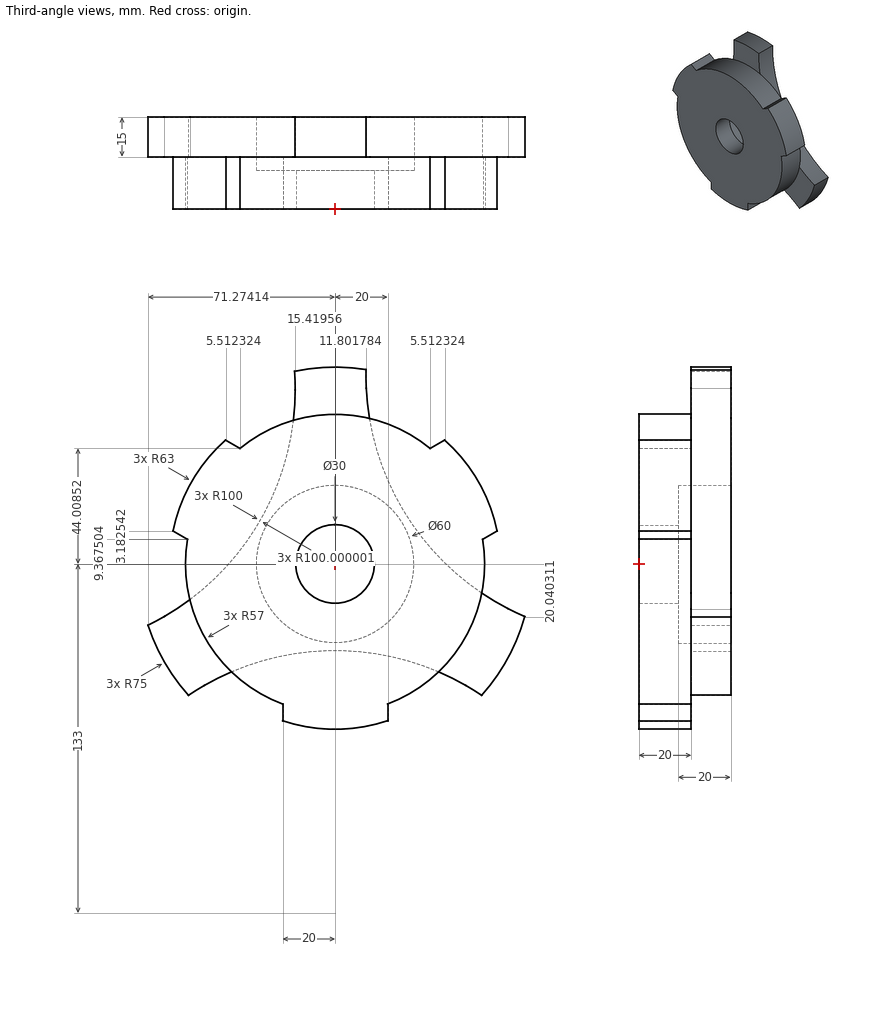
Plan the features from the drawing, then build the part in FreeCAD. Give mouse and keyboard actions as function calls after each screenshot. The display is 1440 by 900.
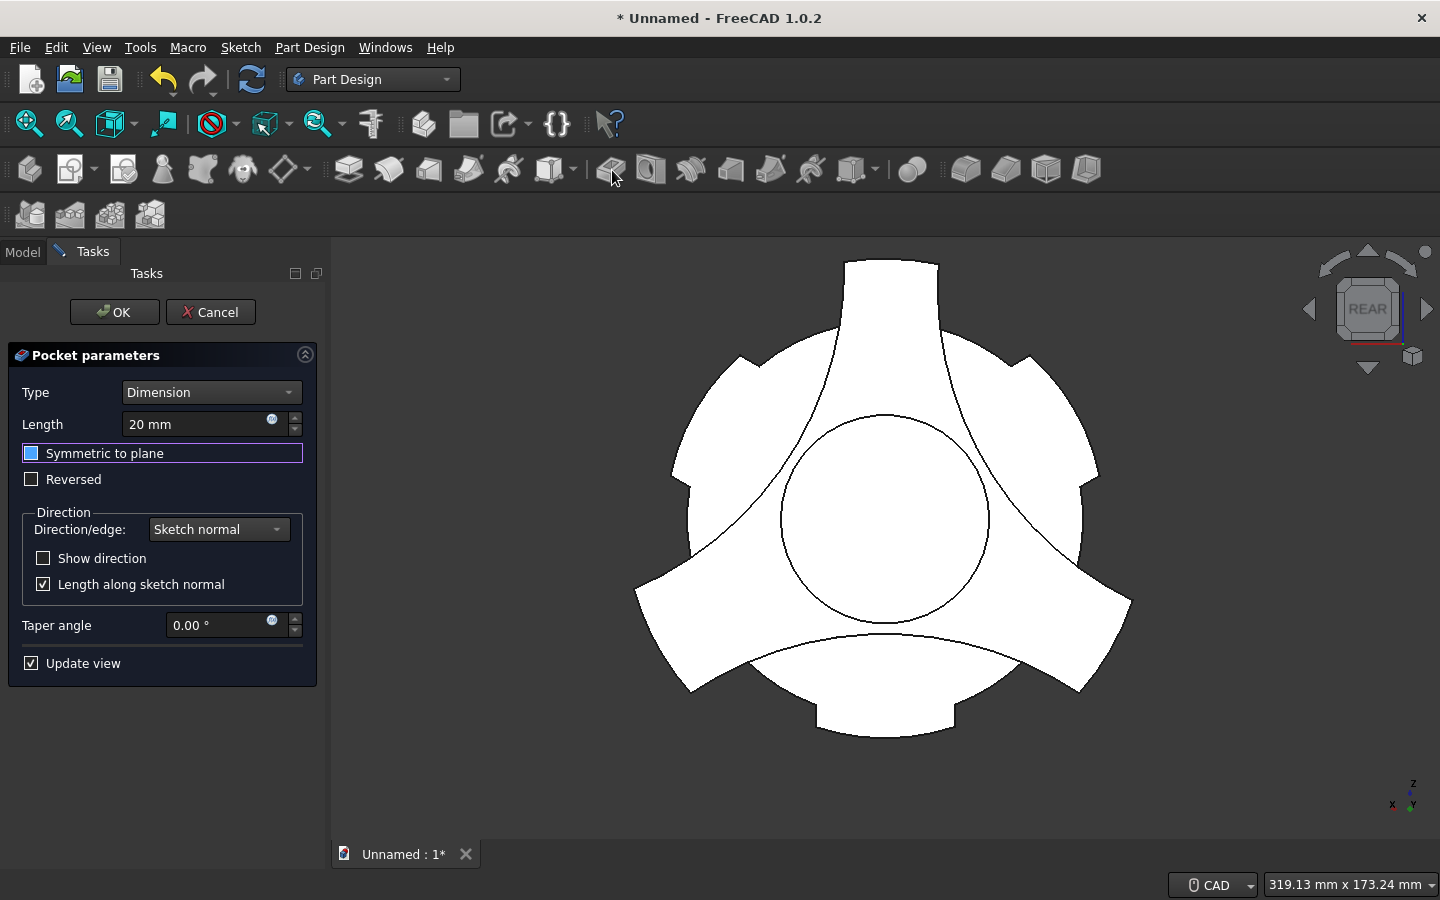
click(115, 312)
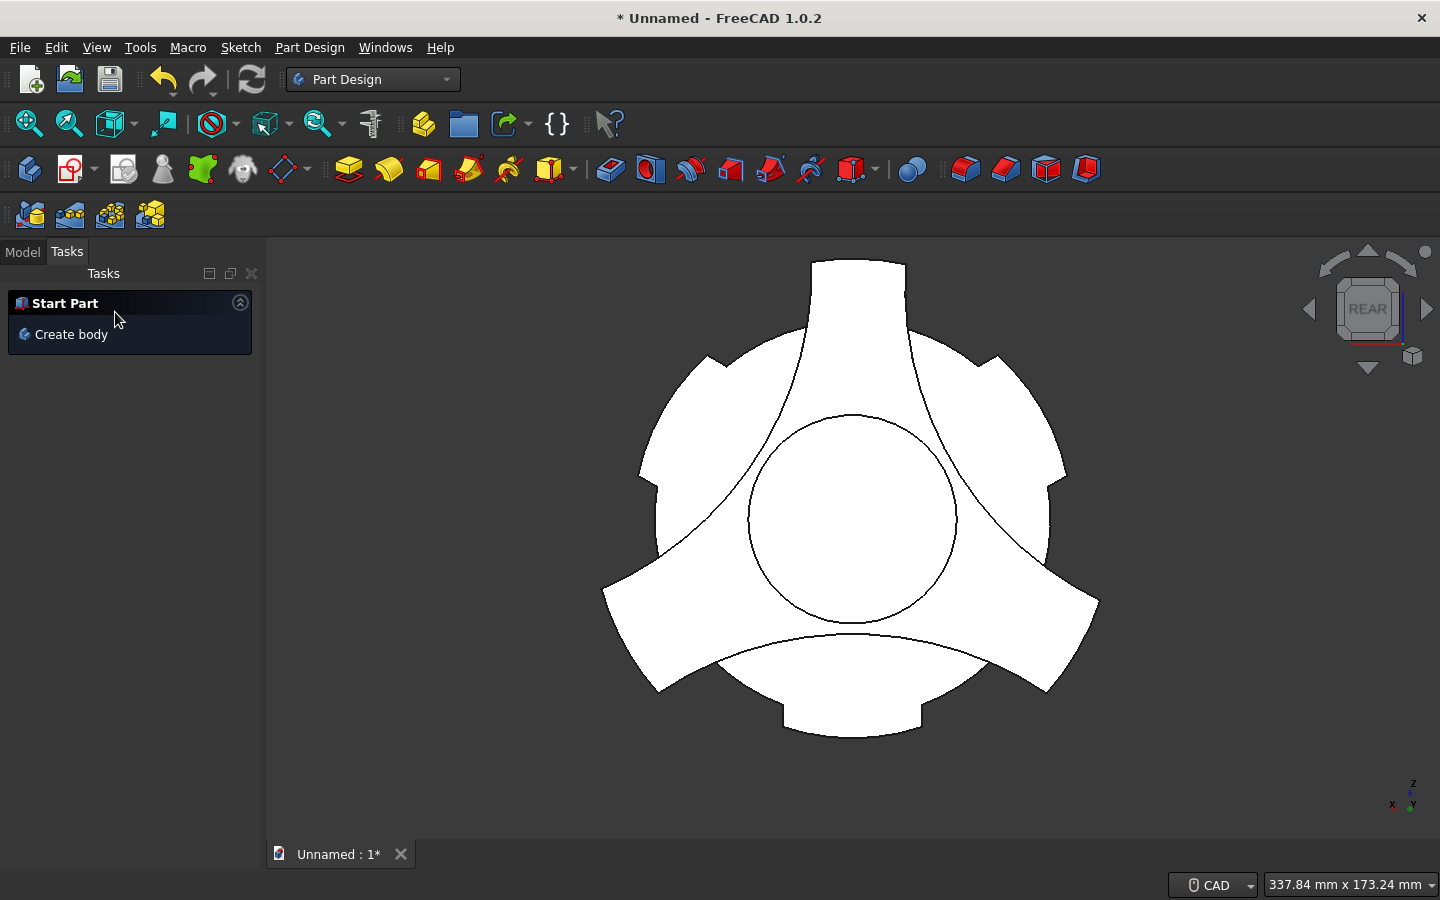
click(853, 518)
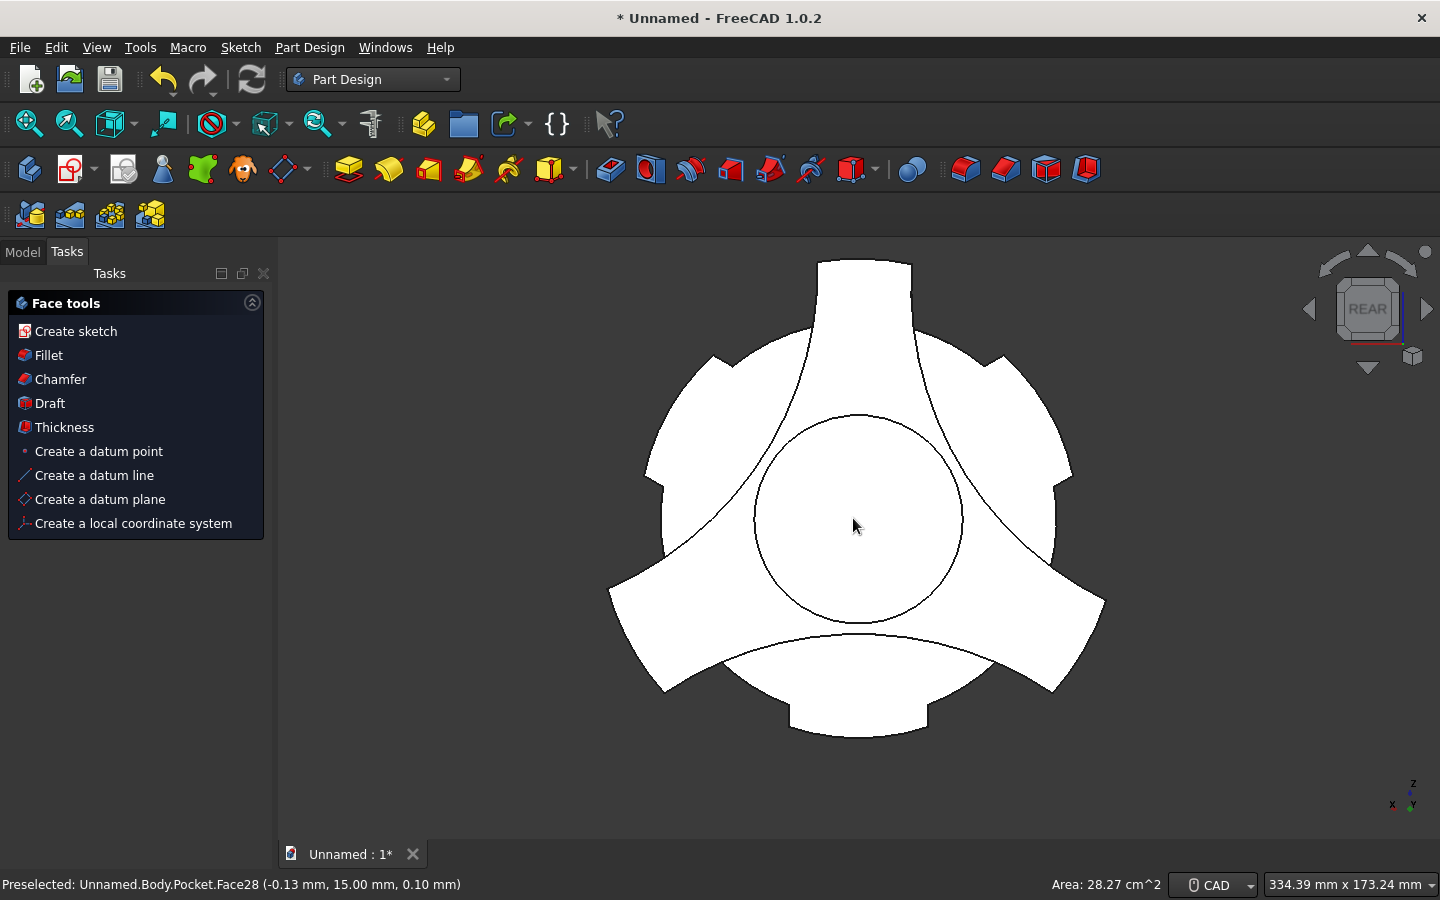
click(70, 170)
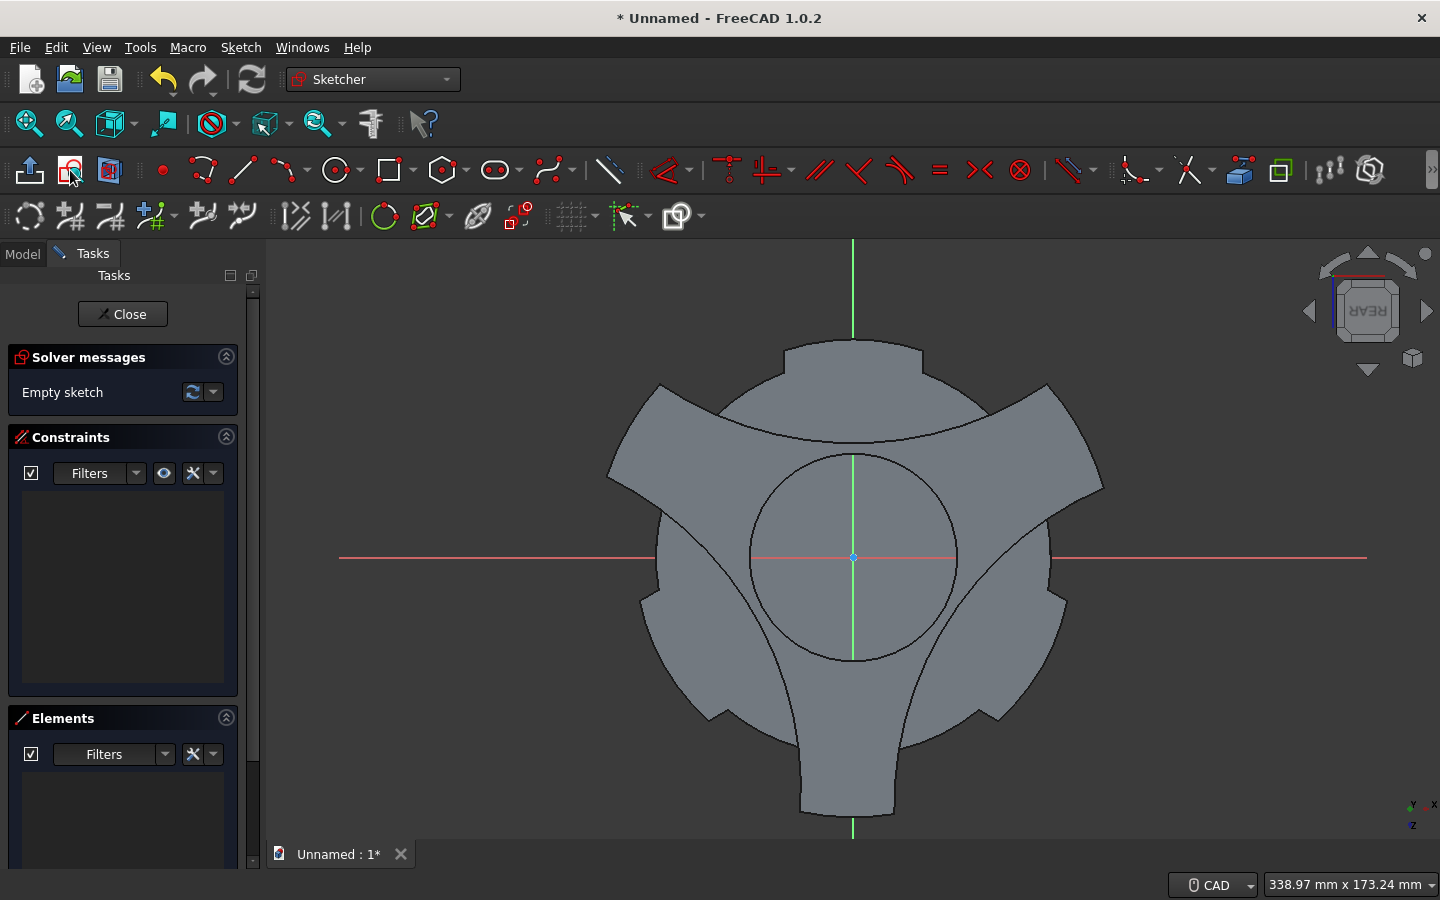
click(110, 170)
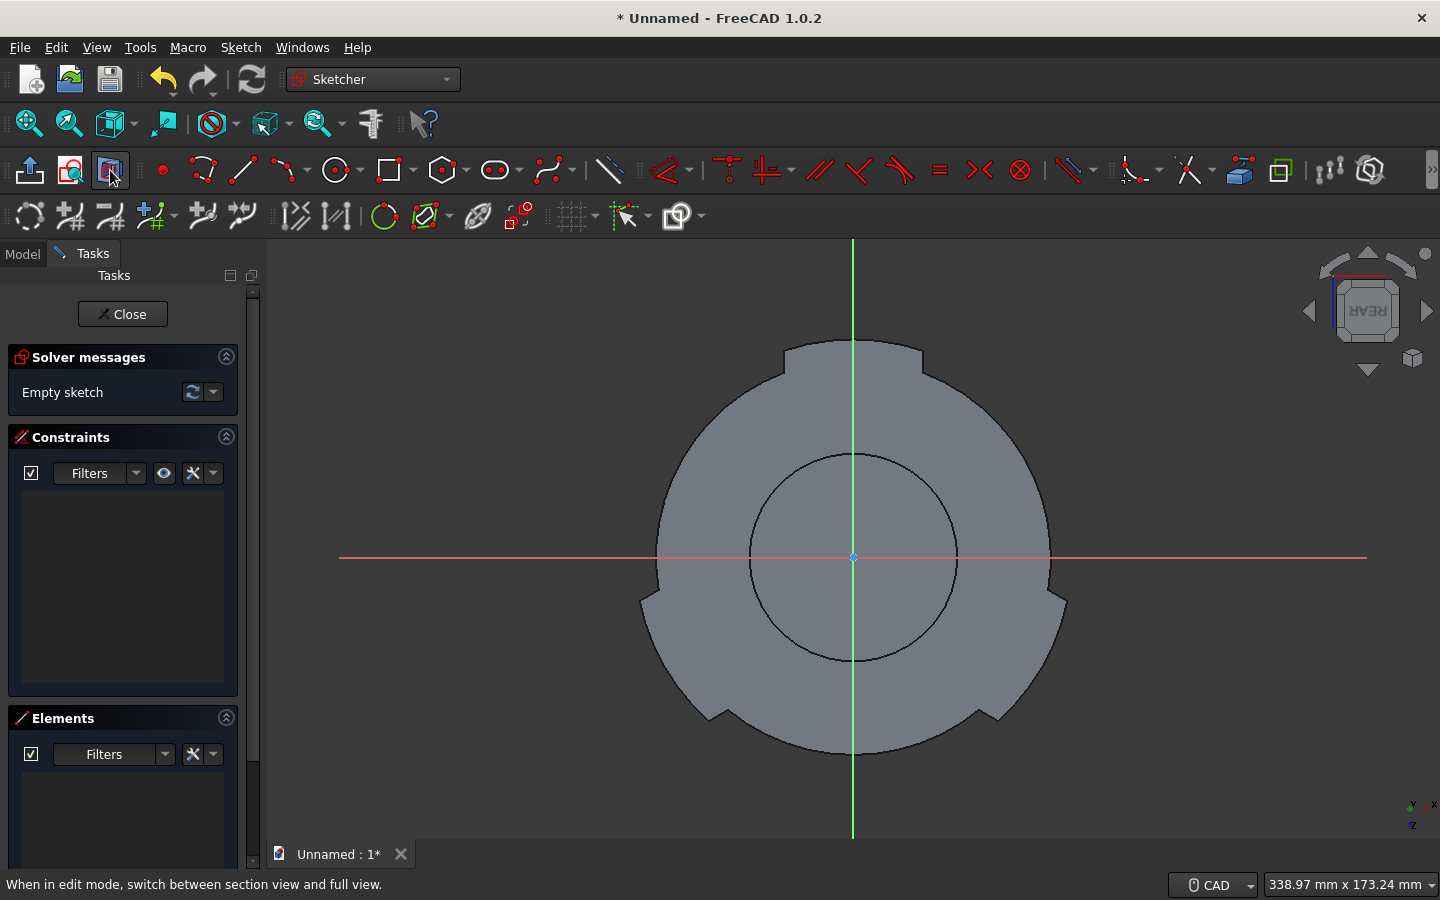
scroll(876, 564, up, 7)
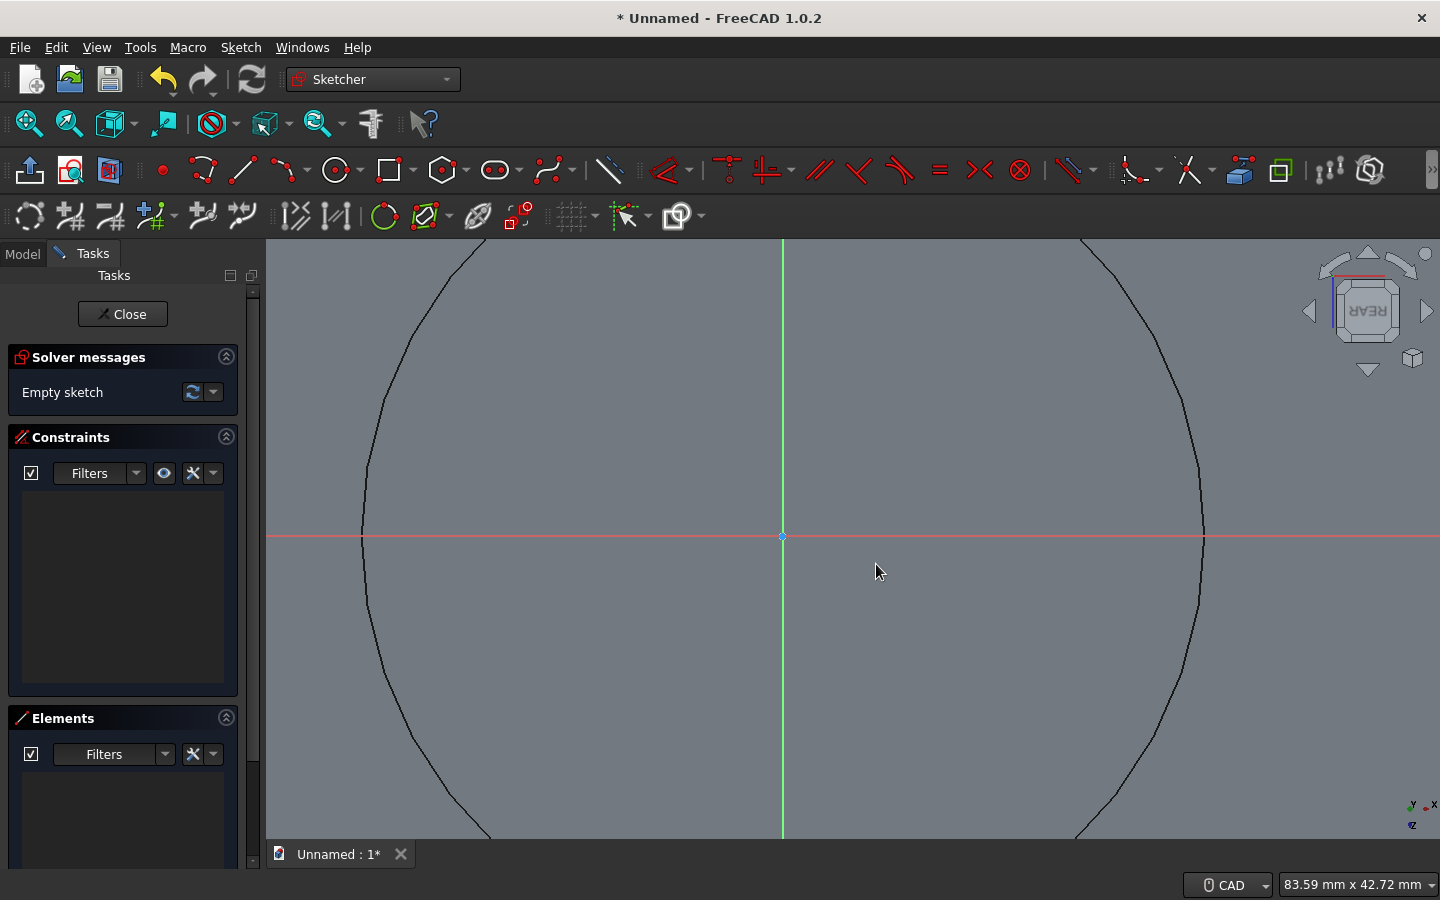
click(336, 170)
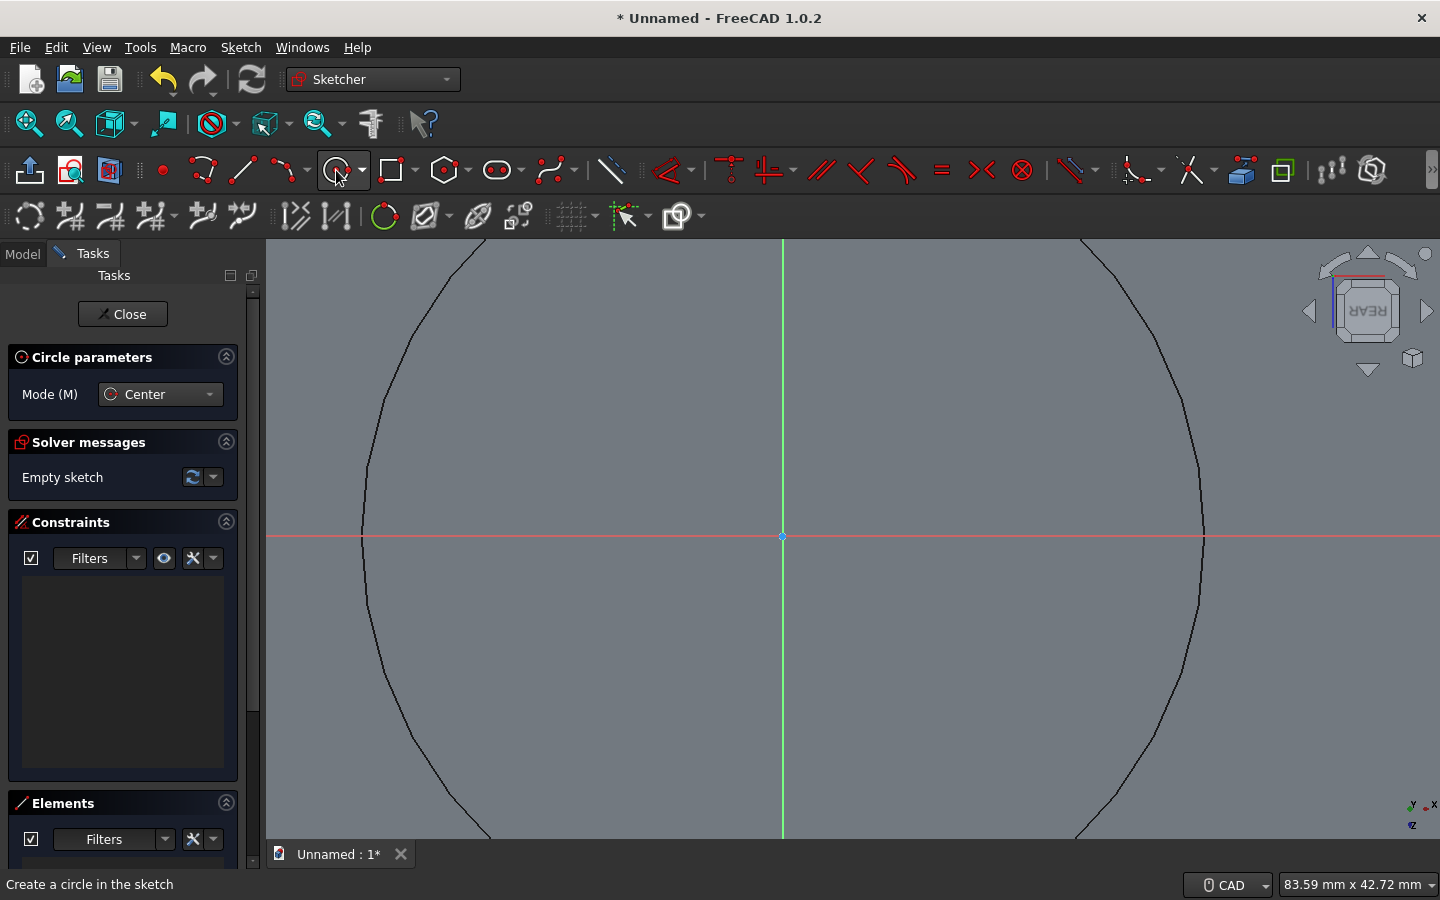
click(783, 536)
move(932, 387)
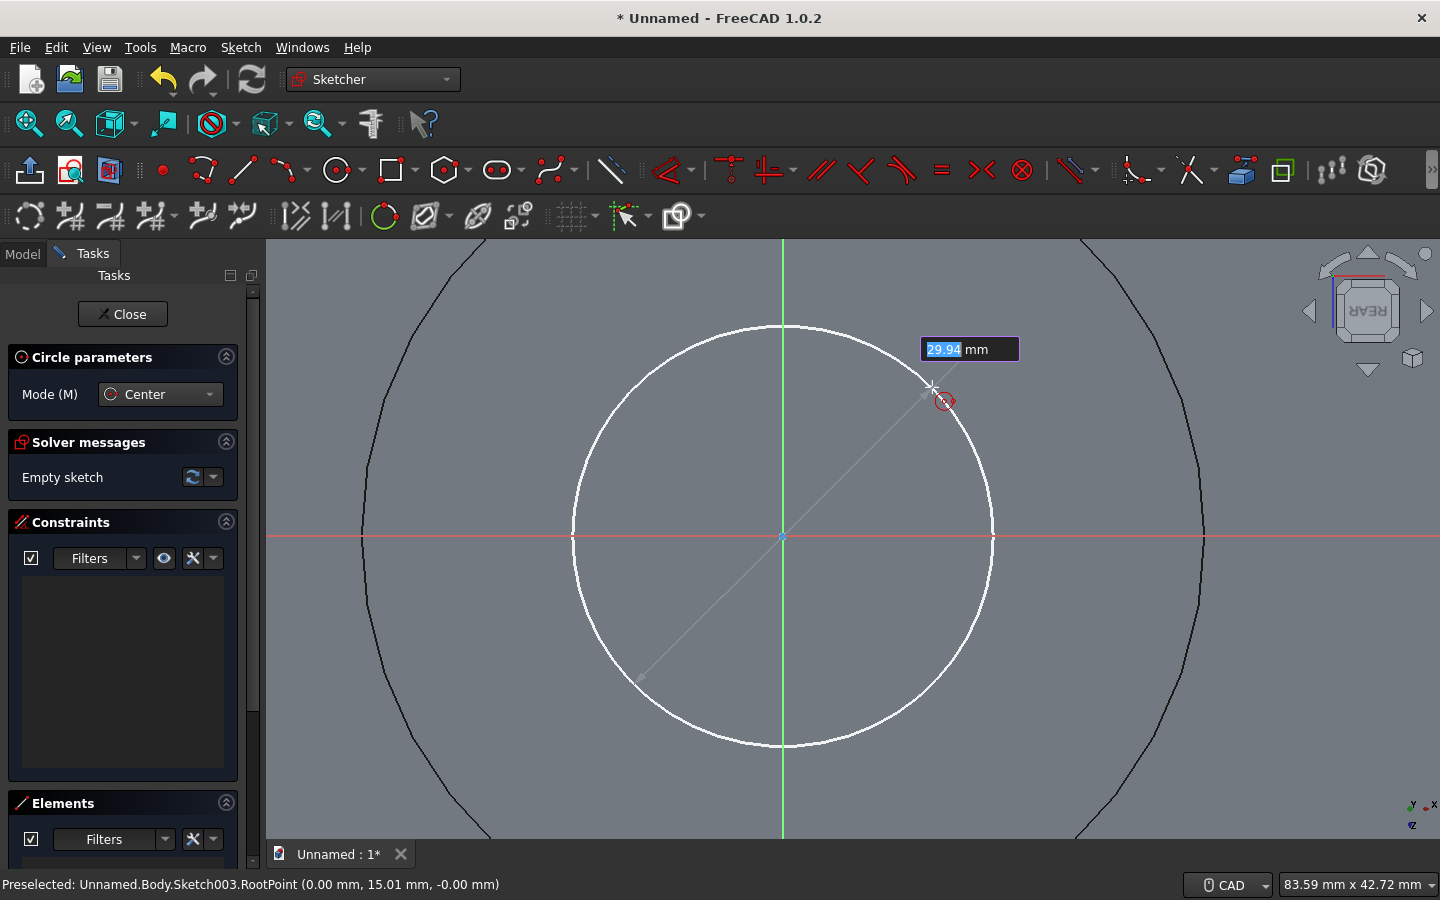
text(30)
key(Return)
key(Escape)